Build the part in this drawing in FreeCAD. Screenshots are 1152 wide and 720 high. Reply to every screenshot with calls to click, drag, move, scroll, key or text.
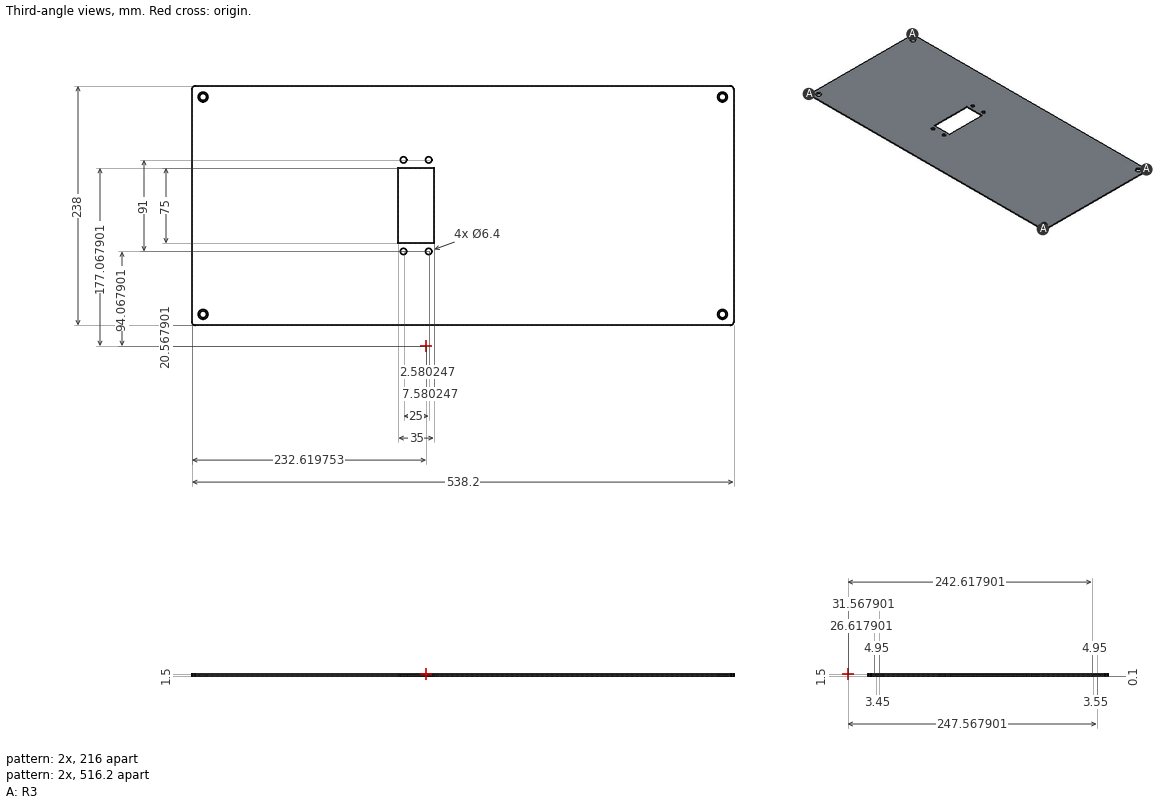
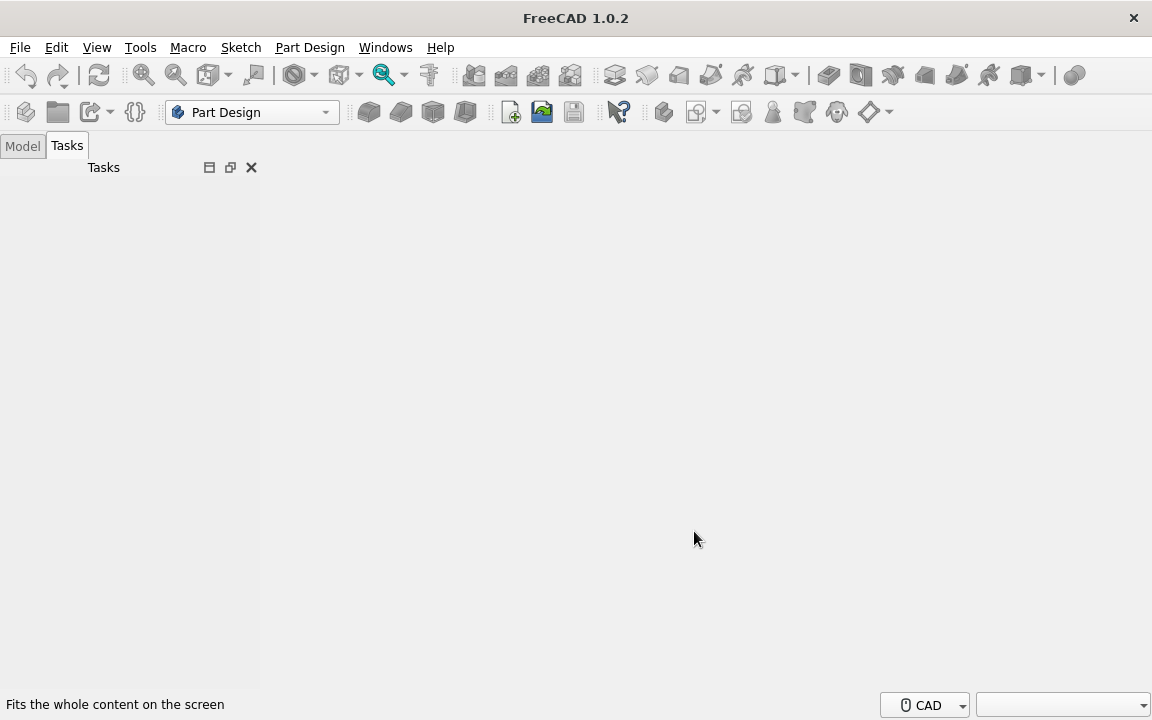
key(ctrl+n)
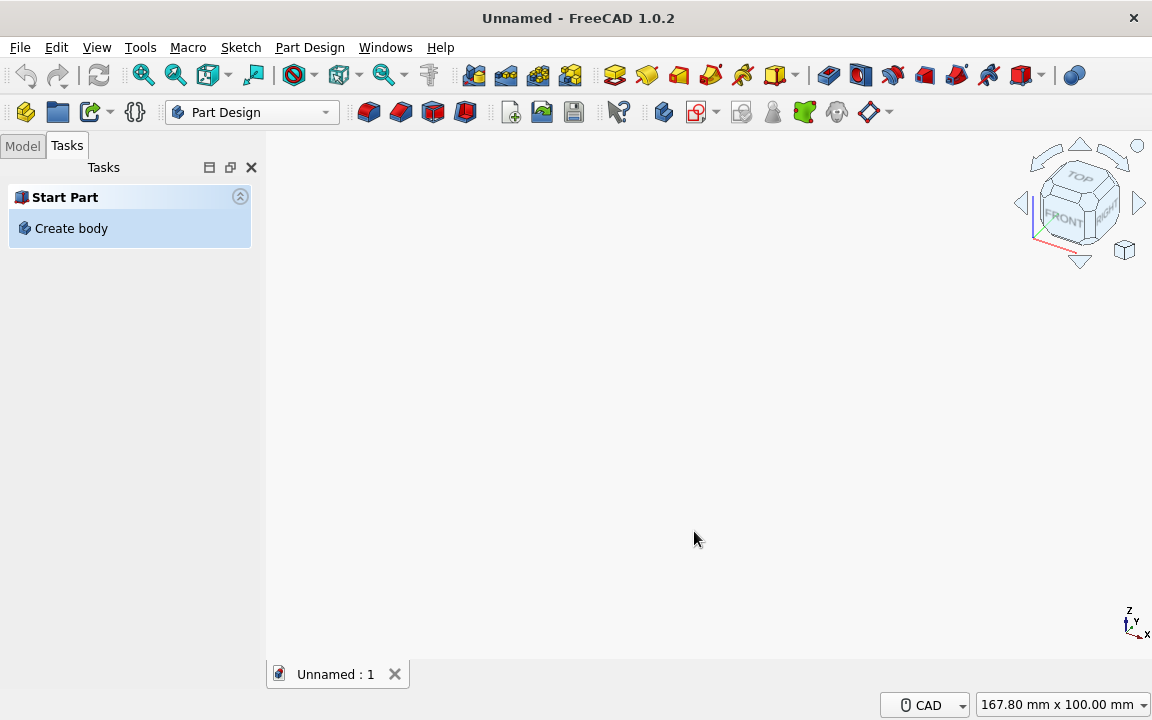
click(696, 112)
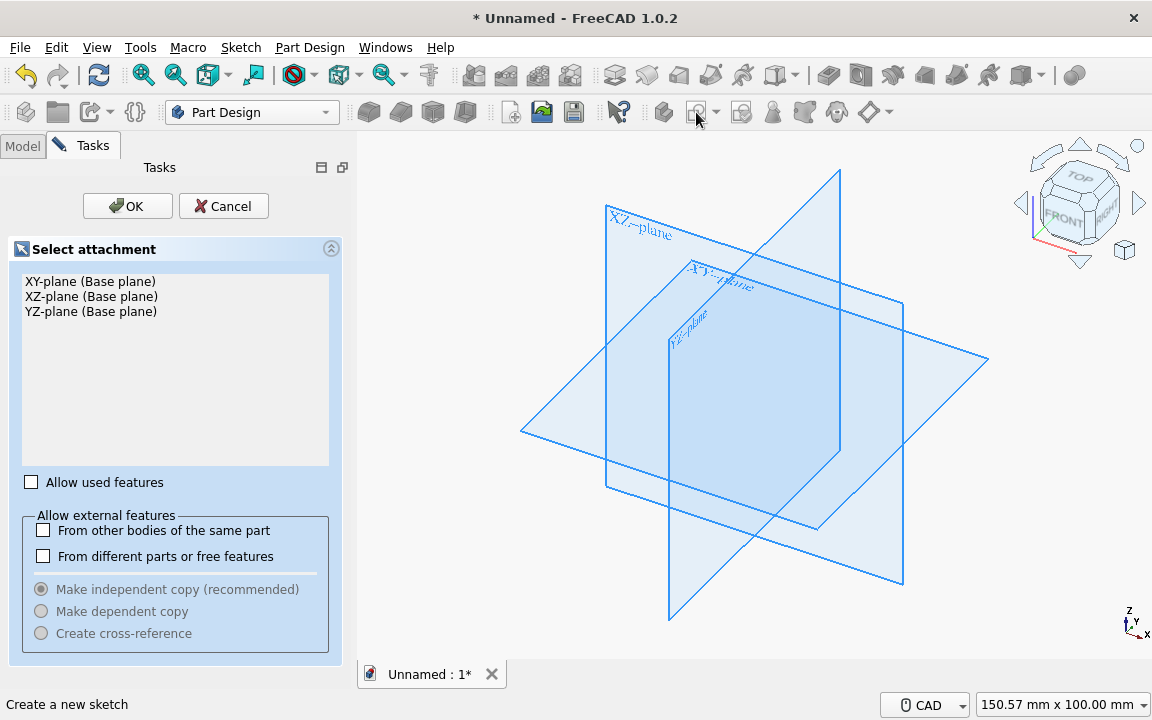
click(82, 282)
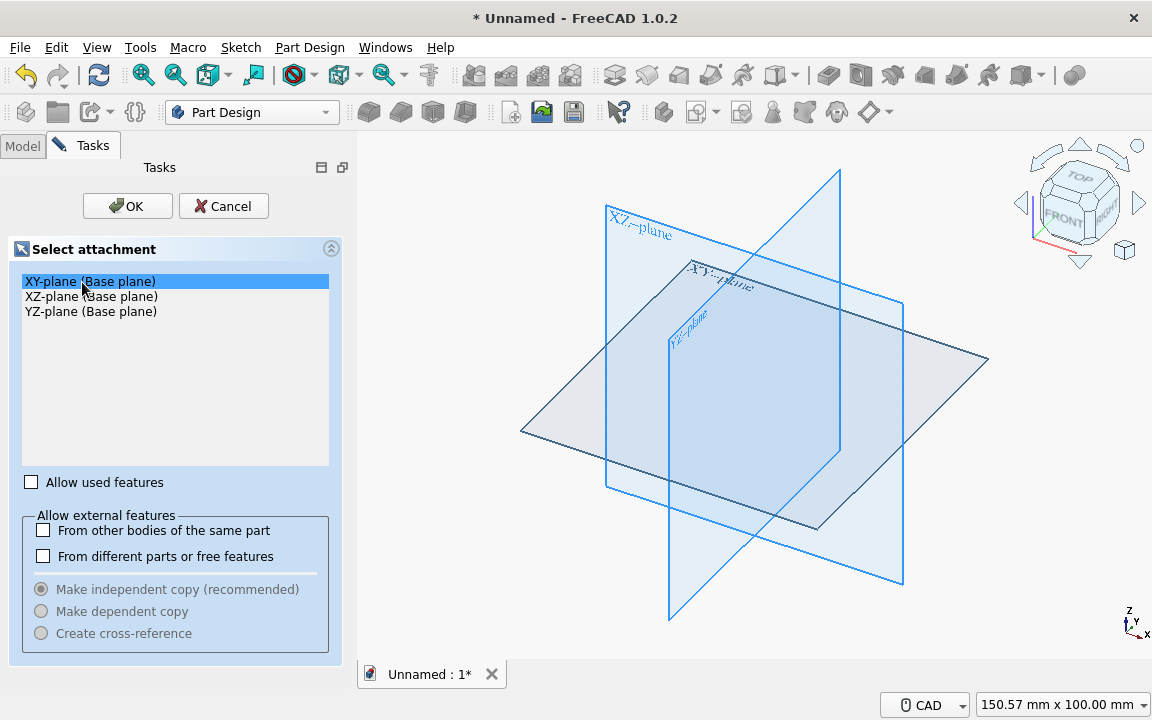
click(128, 206)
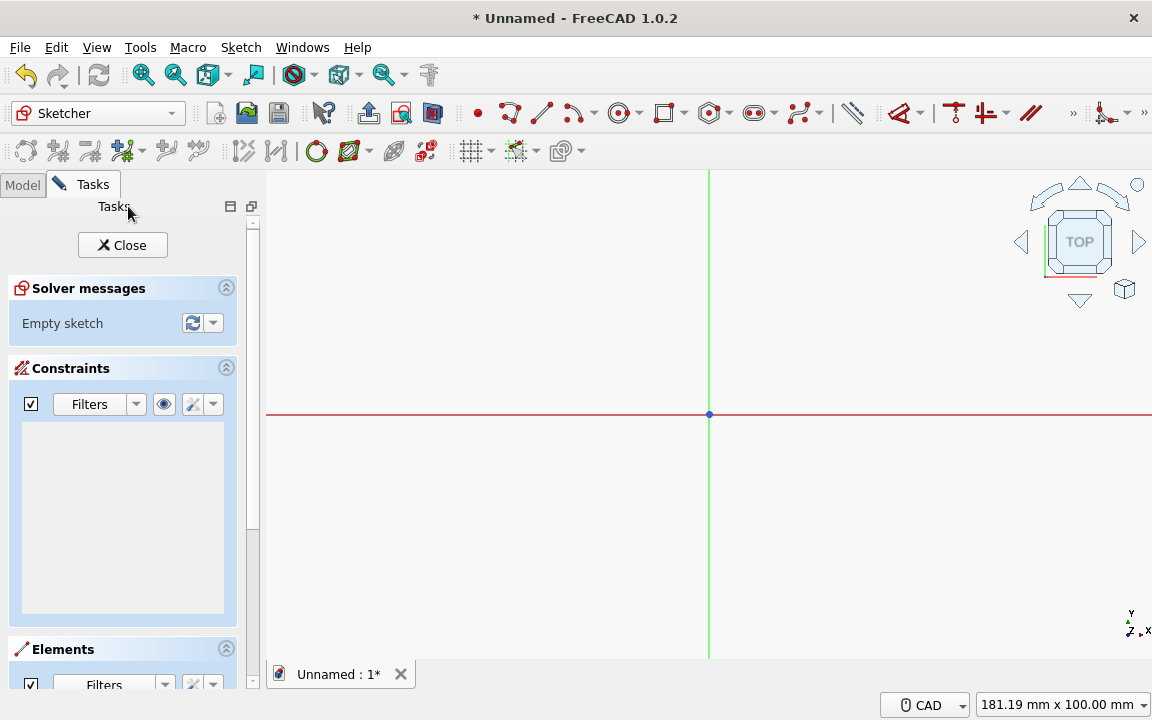
scroll(578, 574, down, 8)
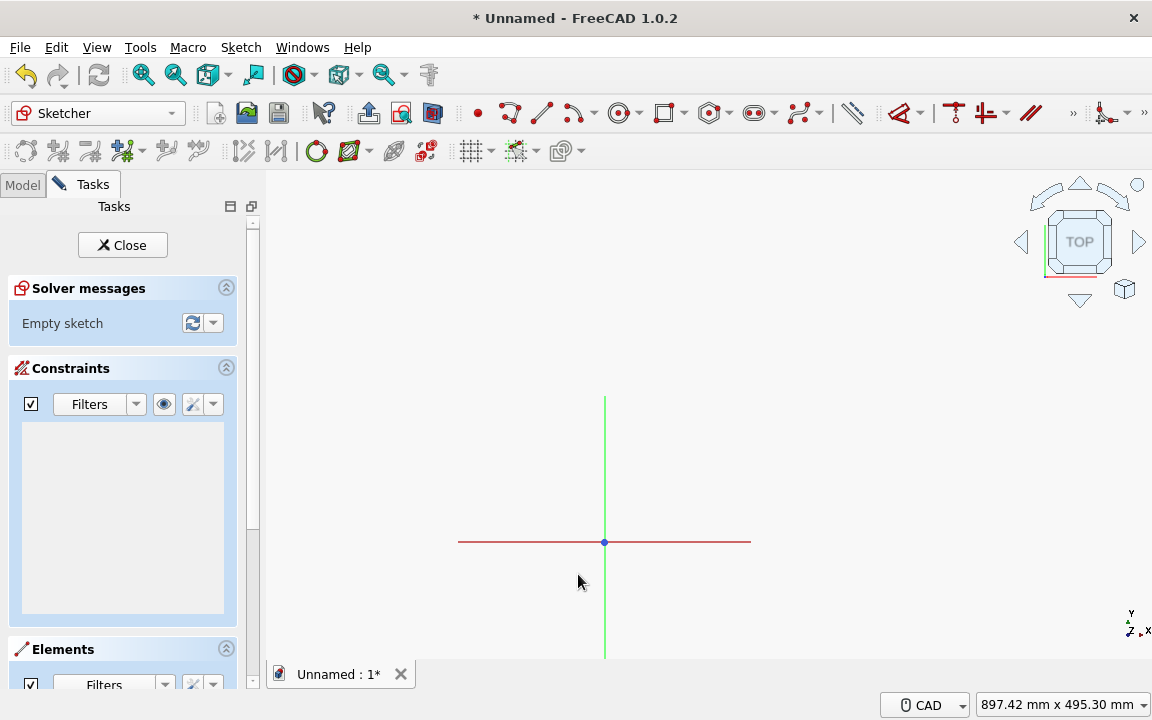
click(664, 114)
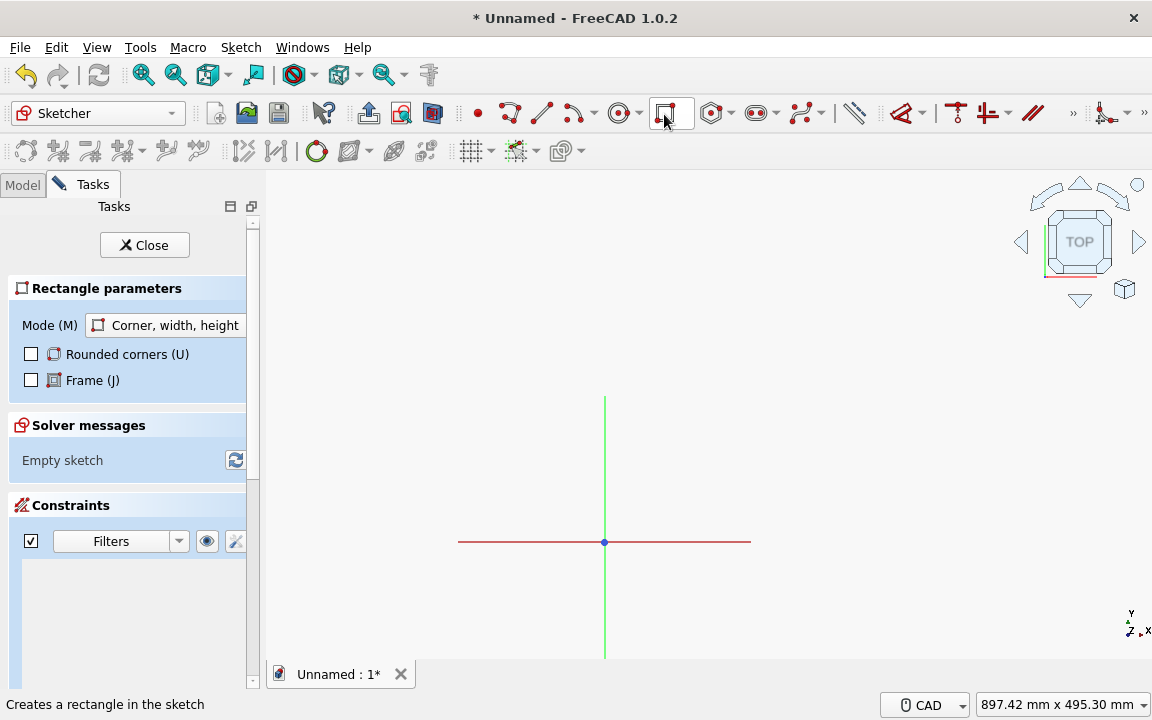
click(375, 287)
click(906, 522)
key(Escape)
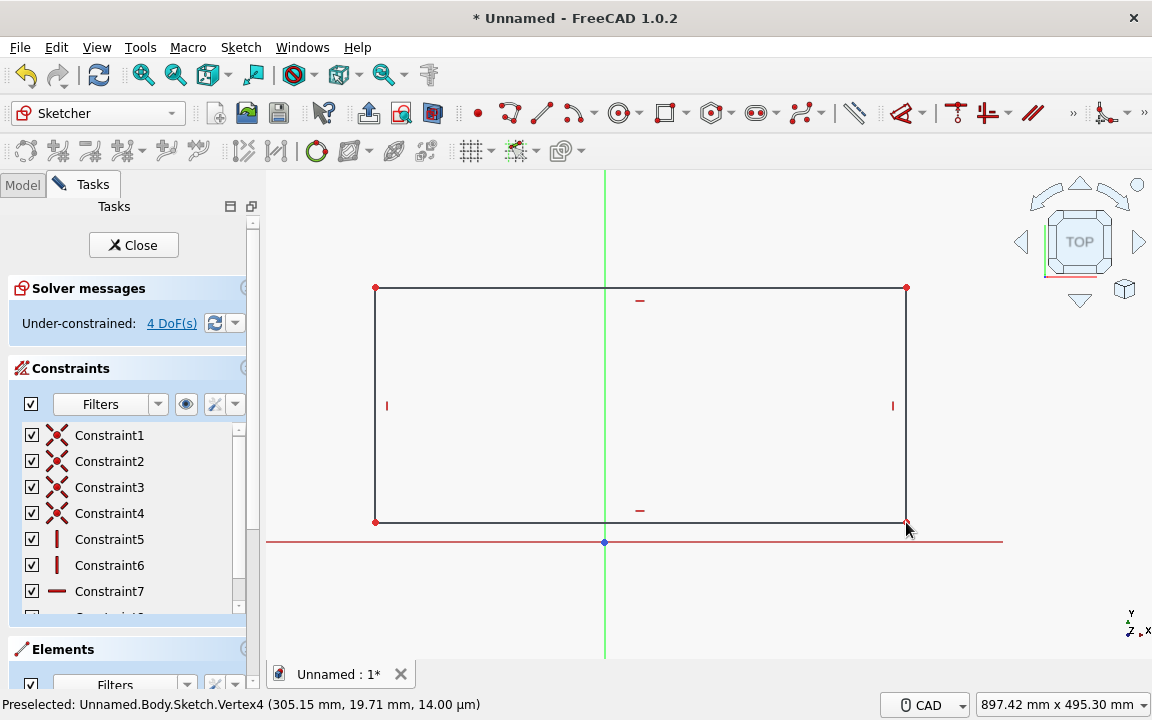
click(902, 114)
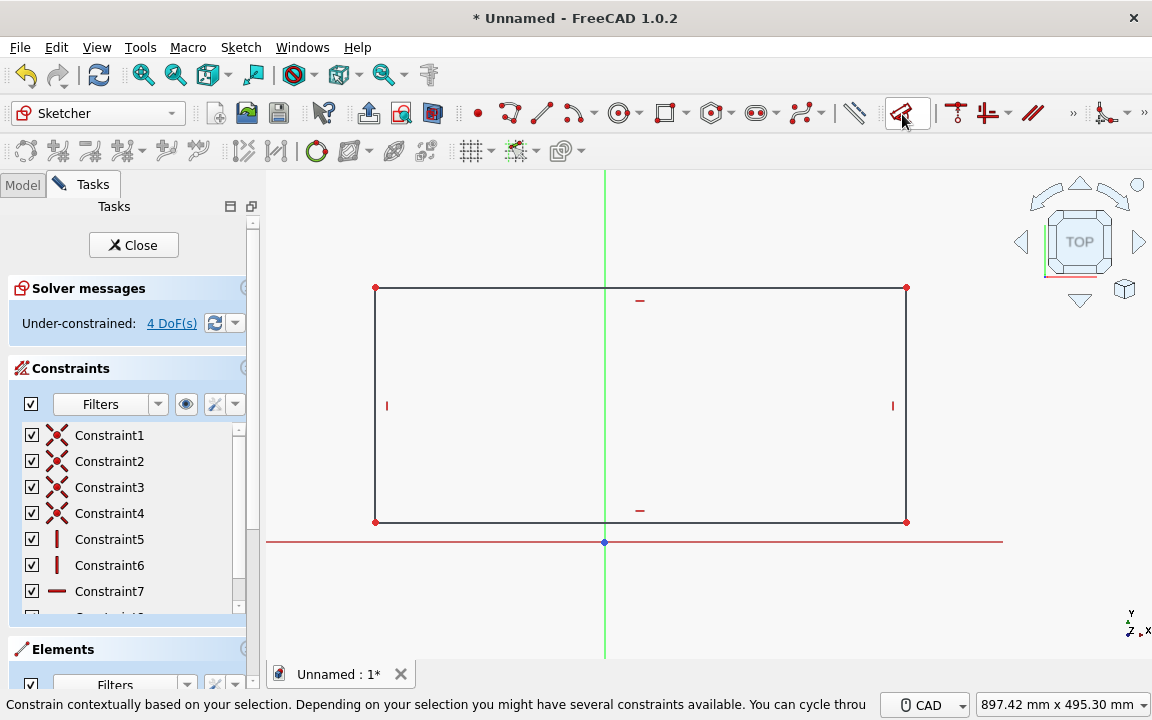
click(375, 359)
click(341, 406)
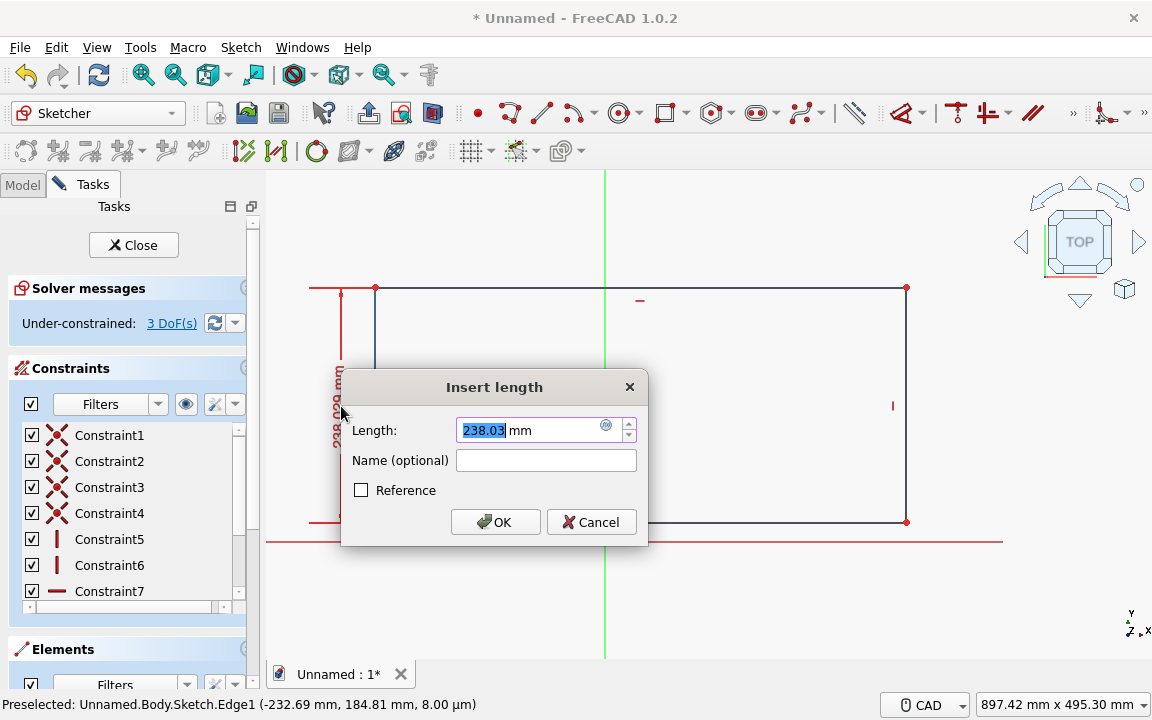
text(238)
key(Return)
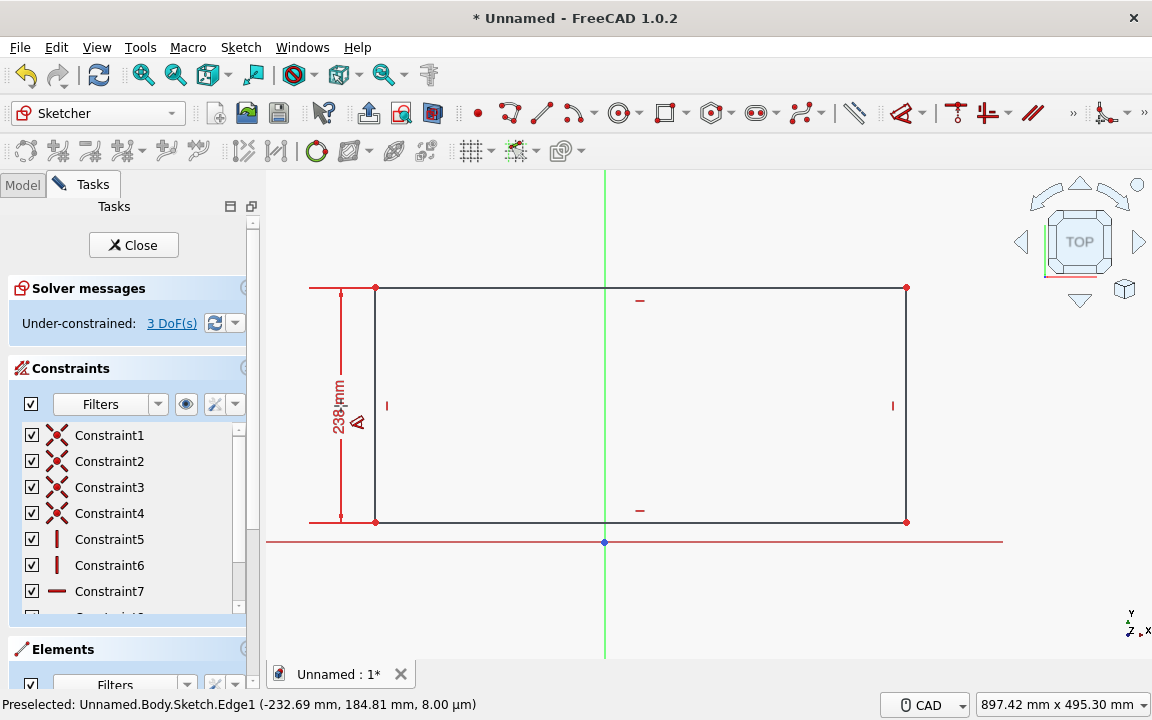
click(534, 523)
click(640, 557)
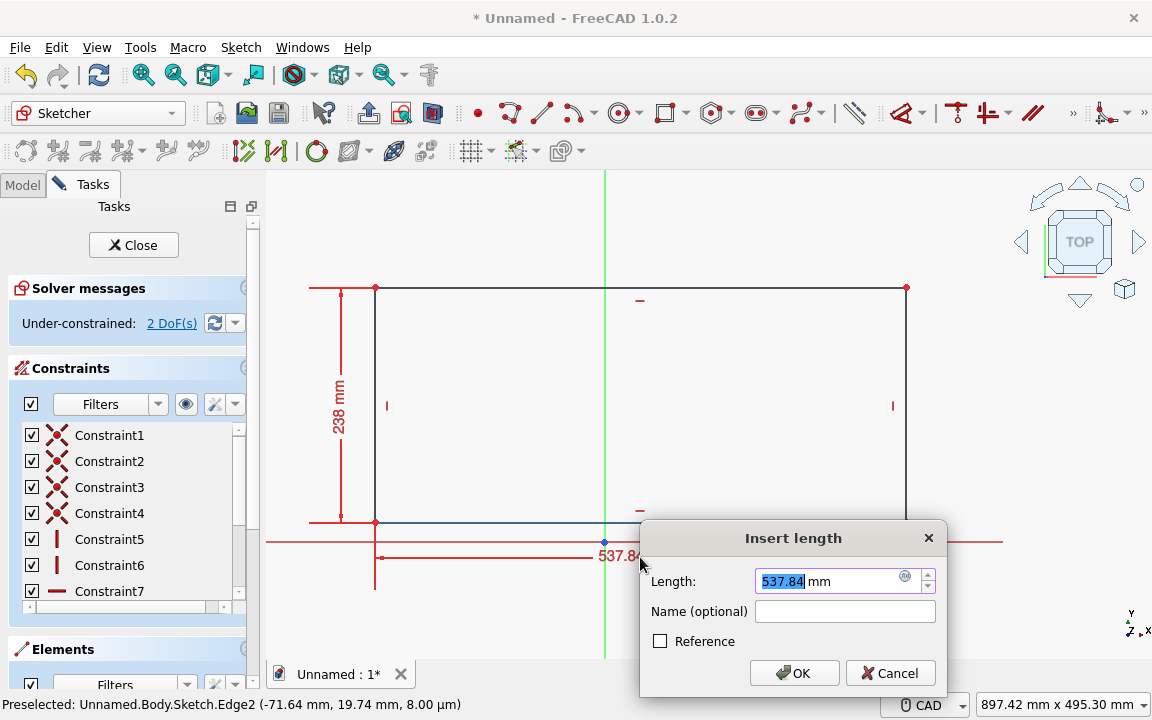
text(538.2)
key(Return)